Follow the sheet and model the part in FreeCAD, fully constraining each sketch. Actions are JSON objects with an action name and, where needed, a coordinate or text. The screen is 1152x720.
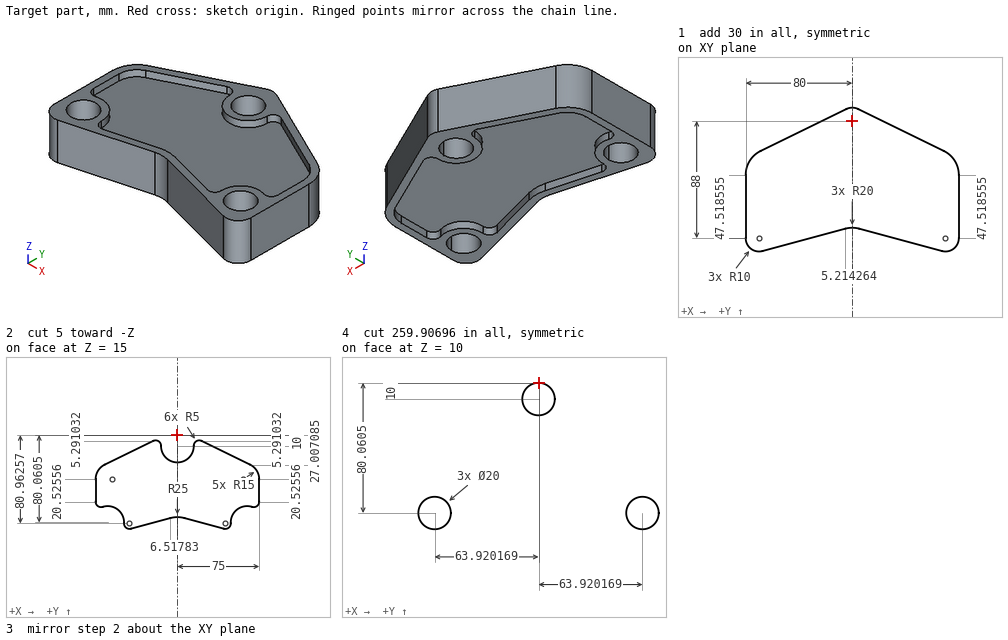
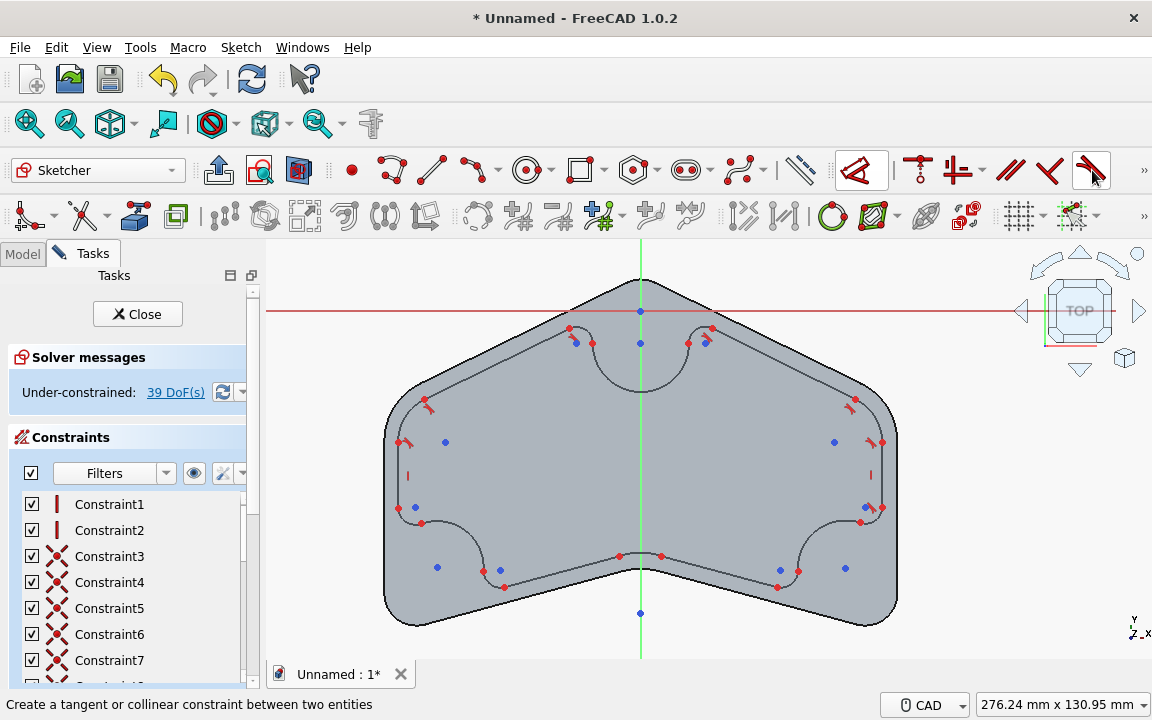
{"action": "left_click", "coordinate": [398, 462]}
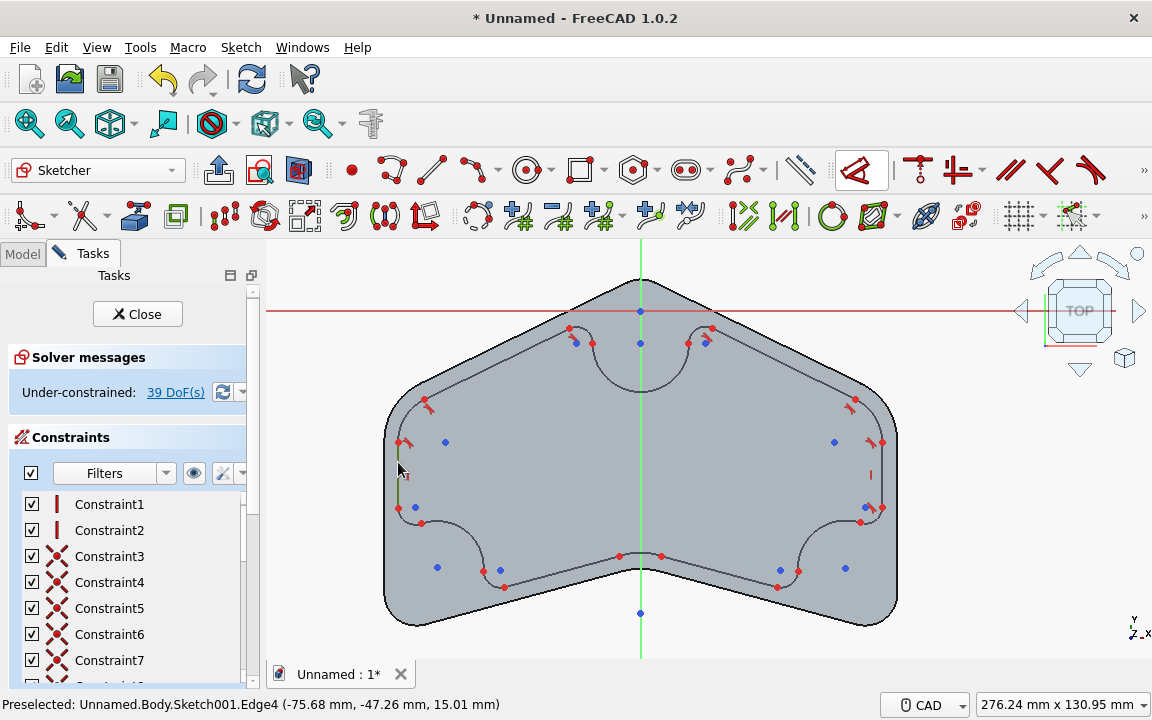
{"action": "scroll", "coordinate": [401, 517], "scroll_direction": "up", "scroll_amount": 2}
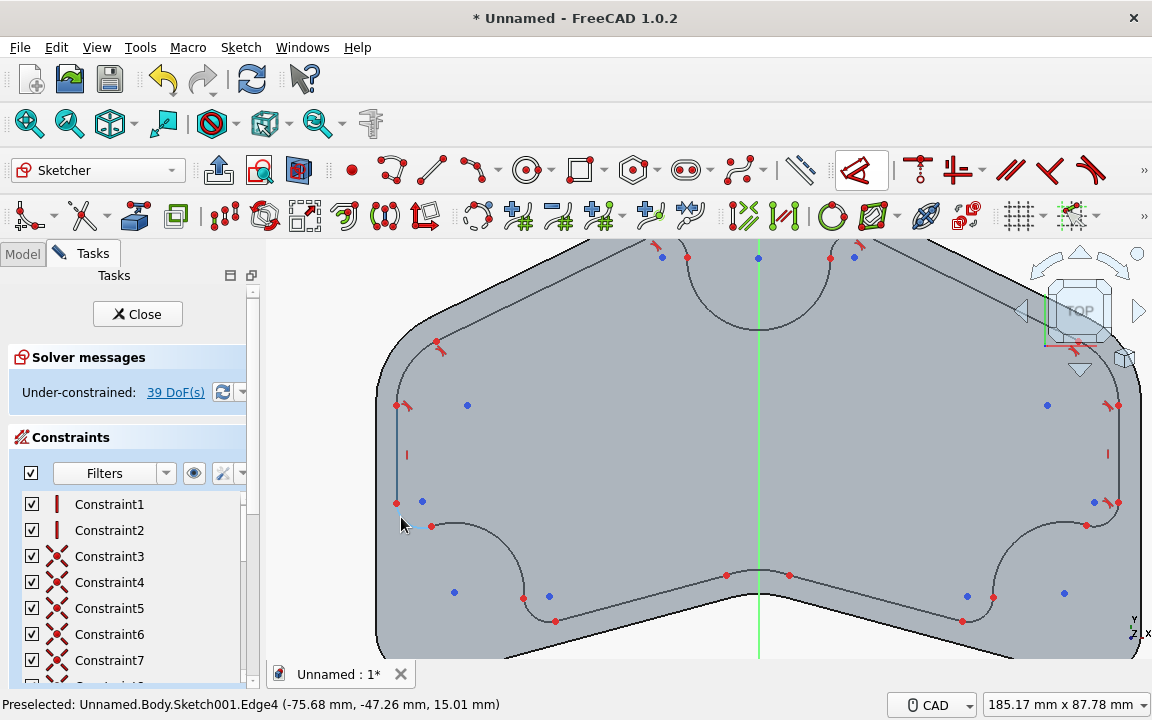
{"action": "left_click", "coordinate": [401, 517]}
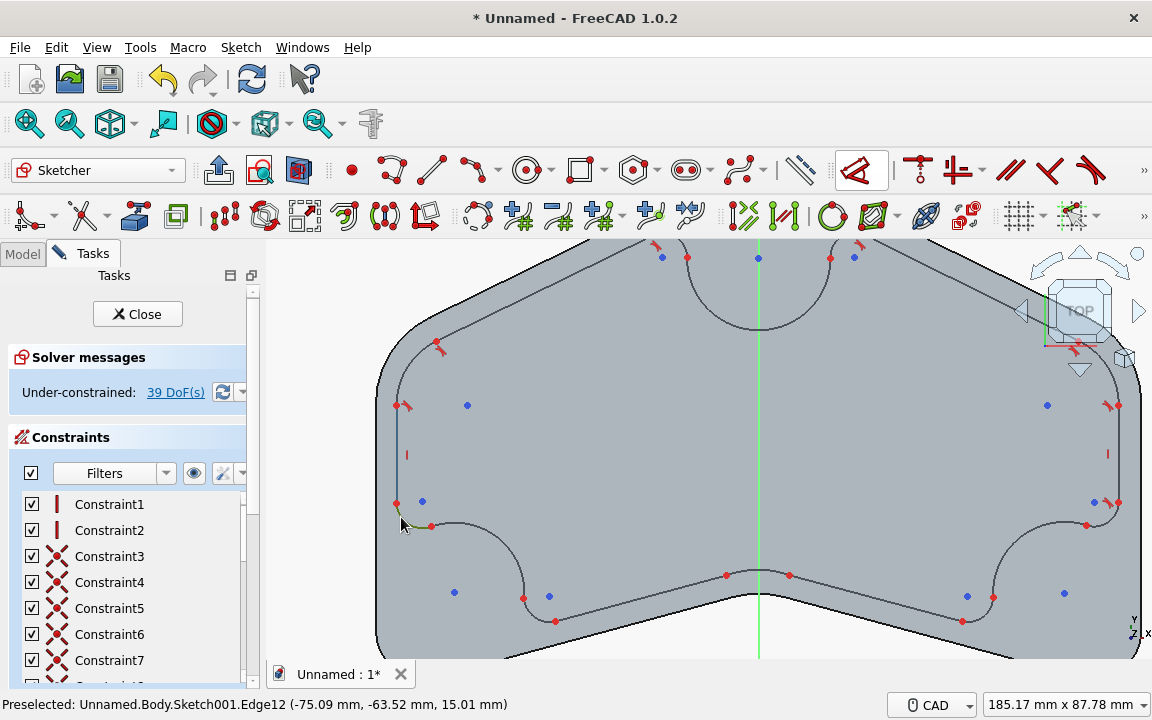
{"action": "left_click", "coordinate": [1092, 170]}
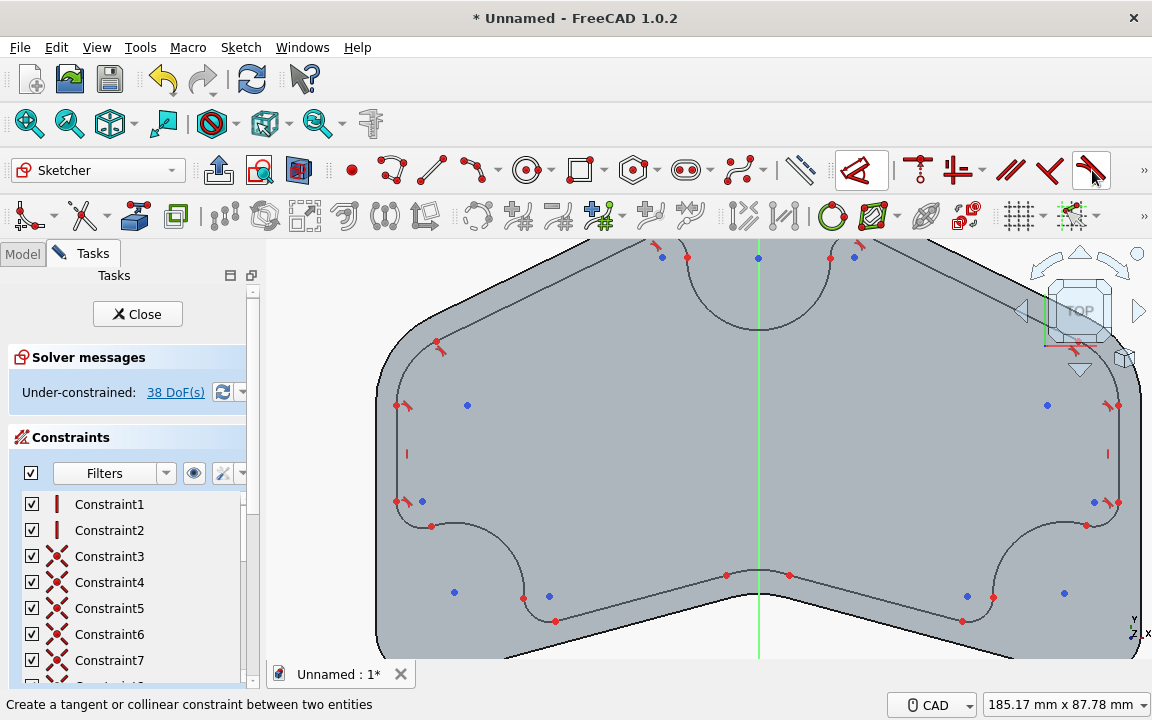
{"action": "left_click", "coordinate": [607, 608]}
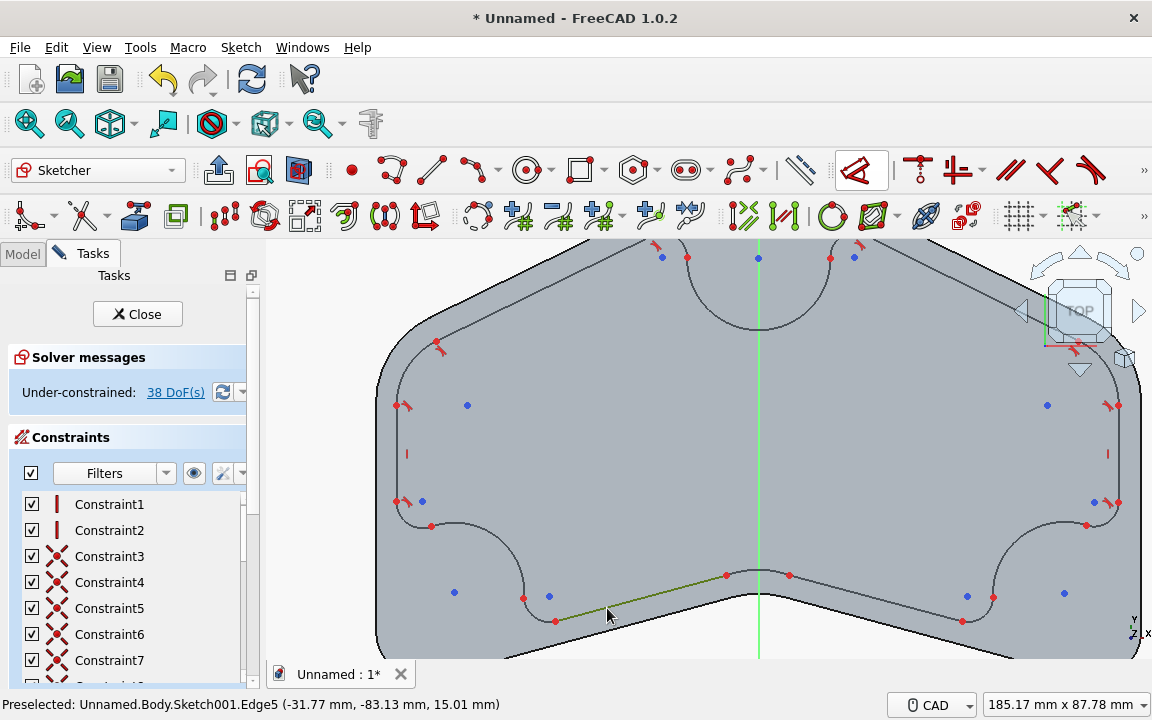
{"action": "left_click", "coordinate": [528, 611]}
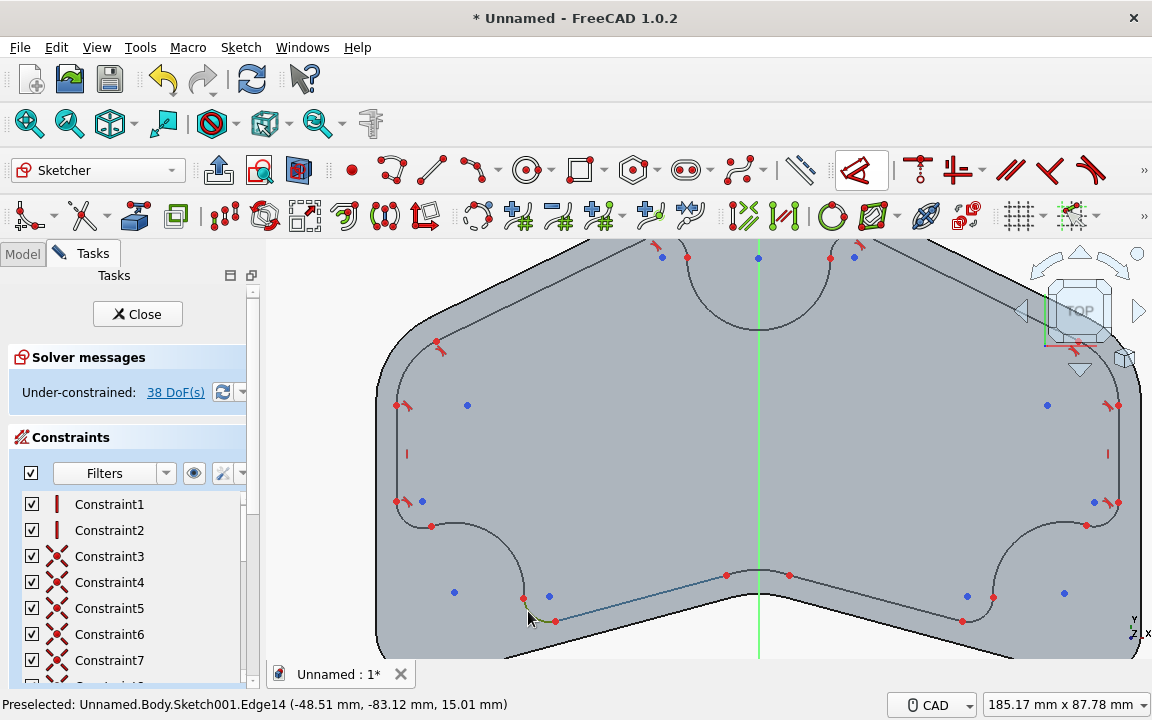
{"action": "left_click", "coordinate": [1092, 170]}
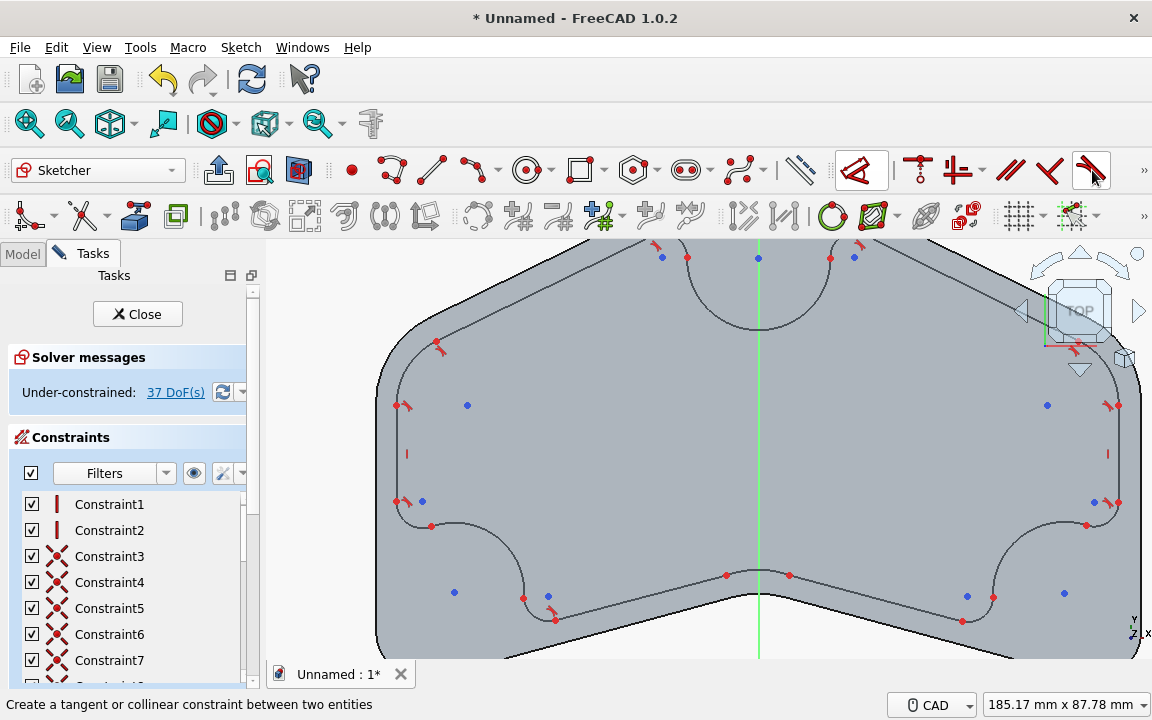
{"action": "left_click", "coordinate": [607, 607]}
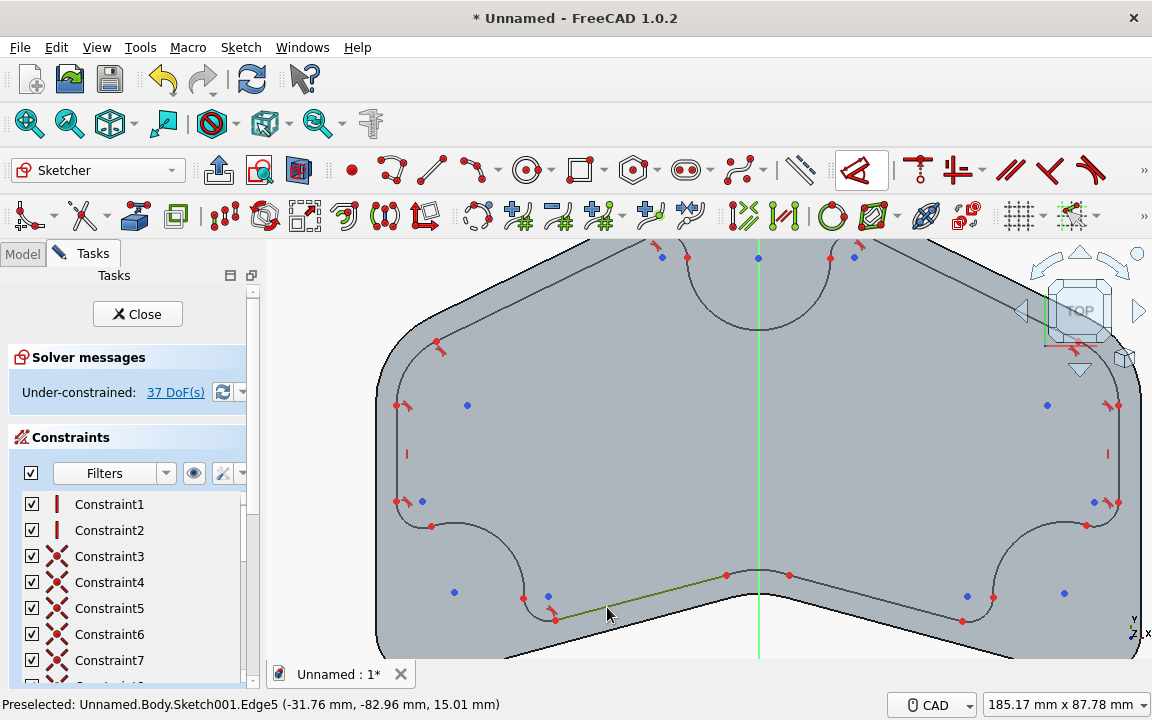
{"action": "left_click", "coordinate": [771, 571]}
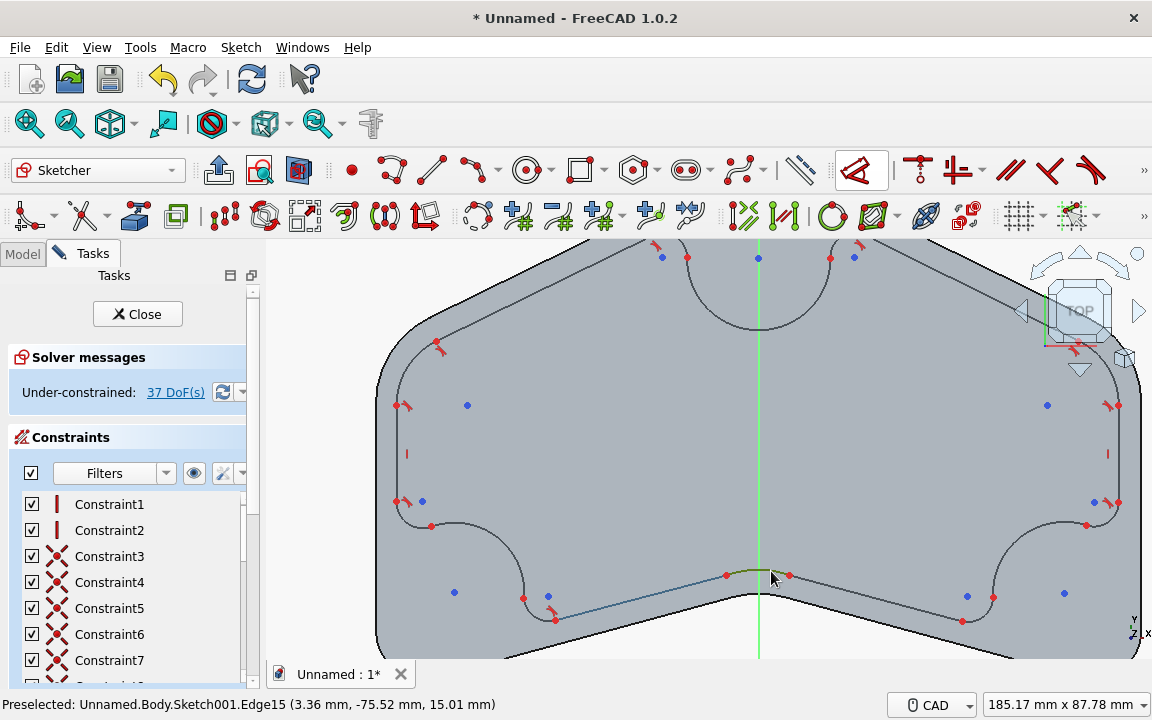
{"action": "left_click", "coordinate": [1092, 170]}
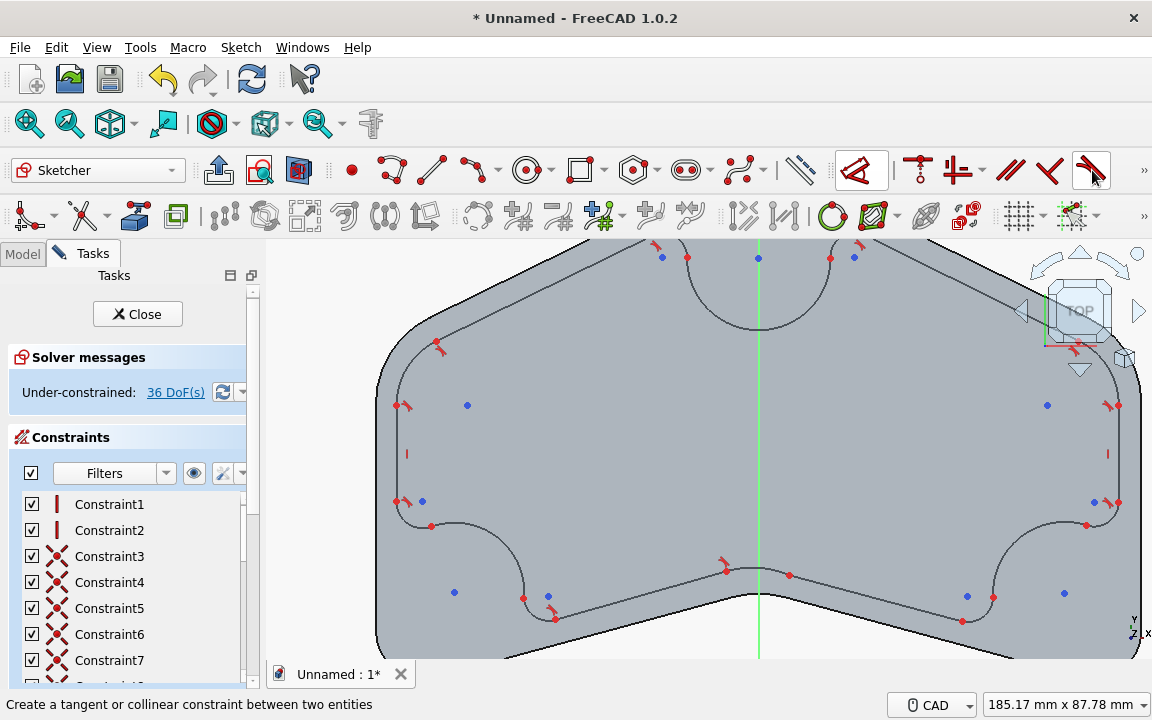
{"action": "left_click", "coordinate": [841, 589]}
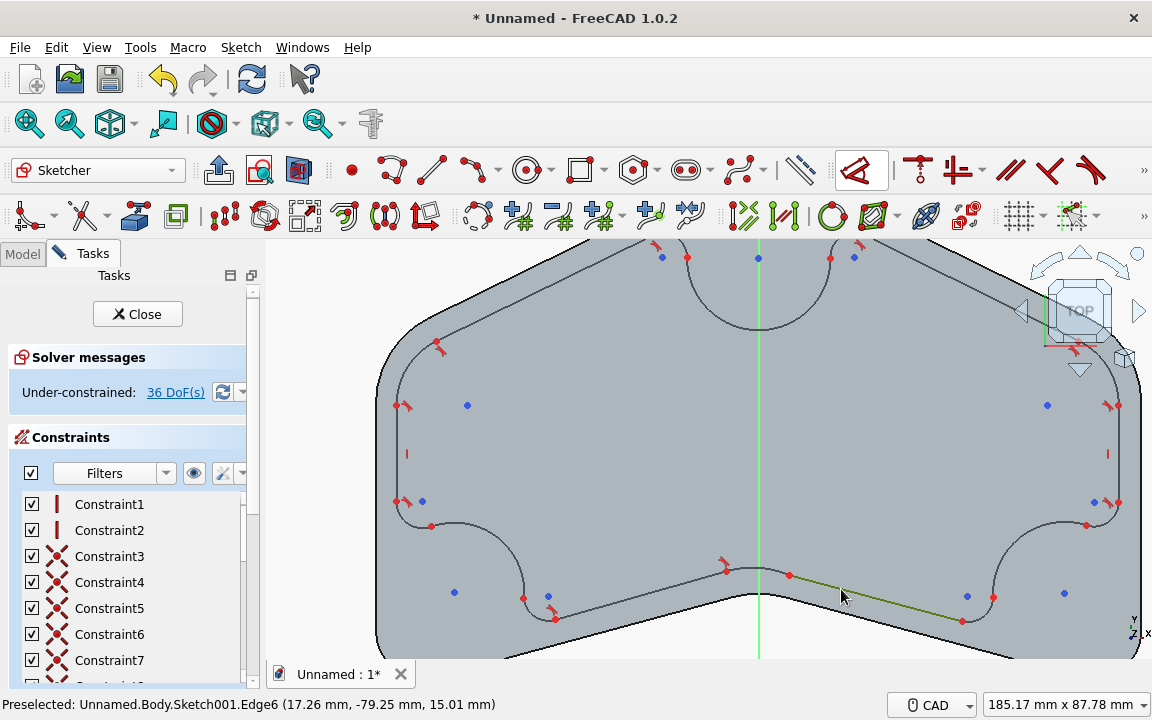
{"action": "left_click", "coordinate": [771, 570]}